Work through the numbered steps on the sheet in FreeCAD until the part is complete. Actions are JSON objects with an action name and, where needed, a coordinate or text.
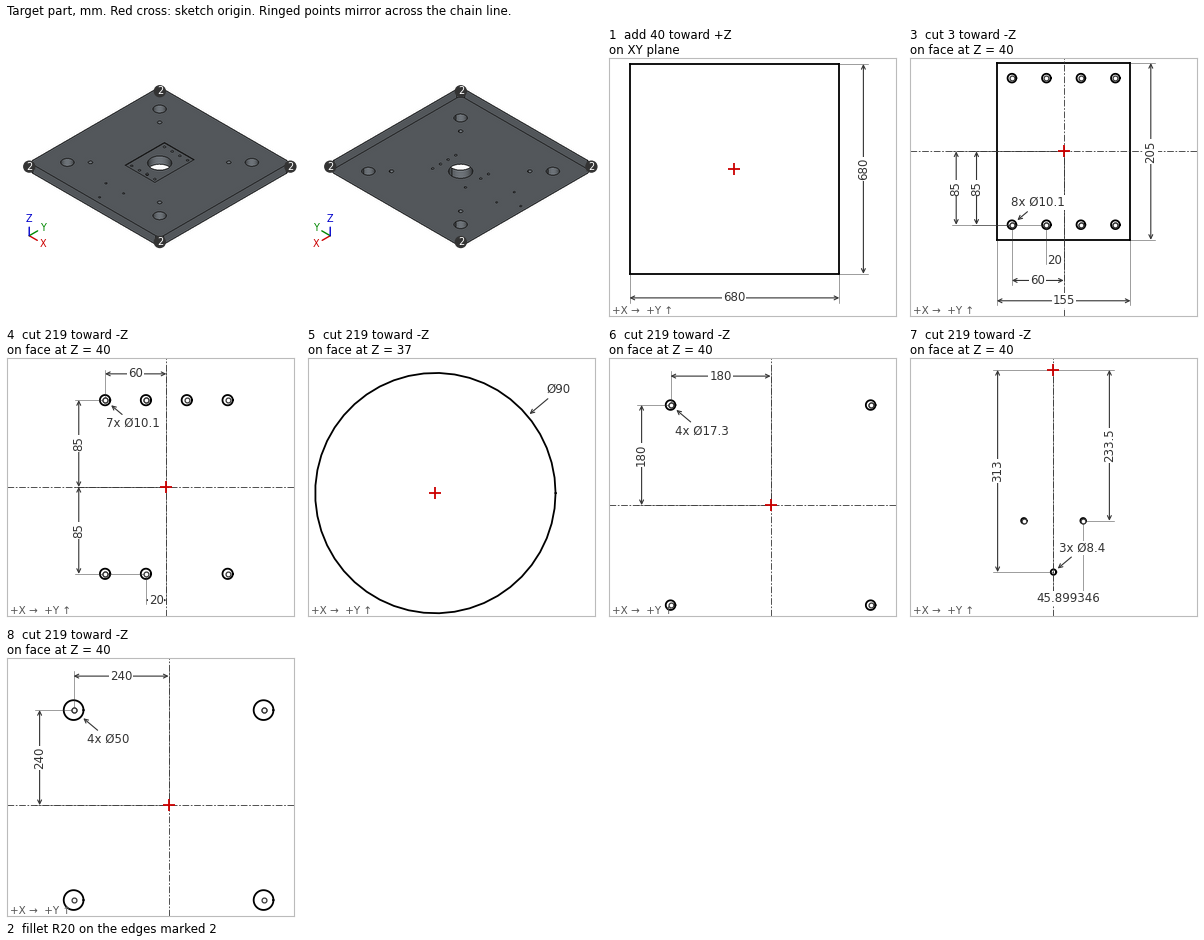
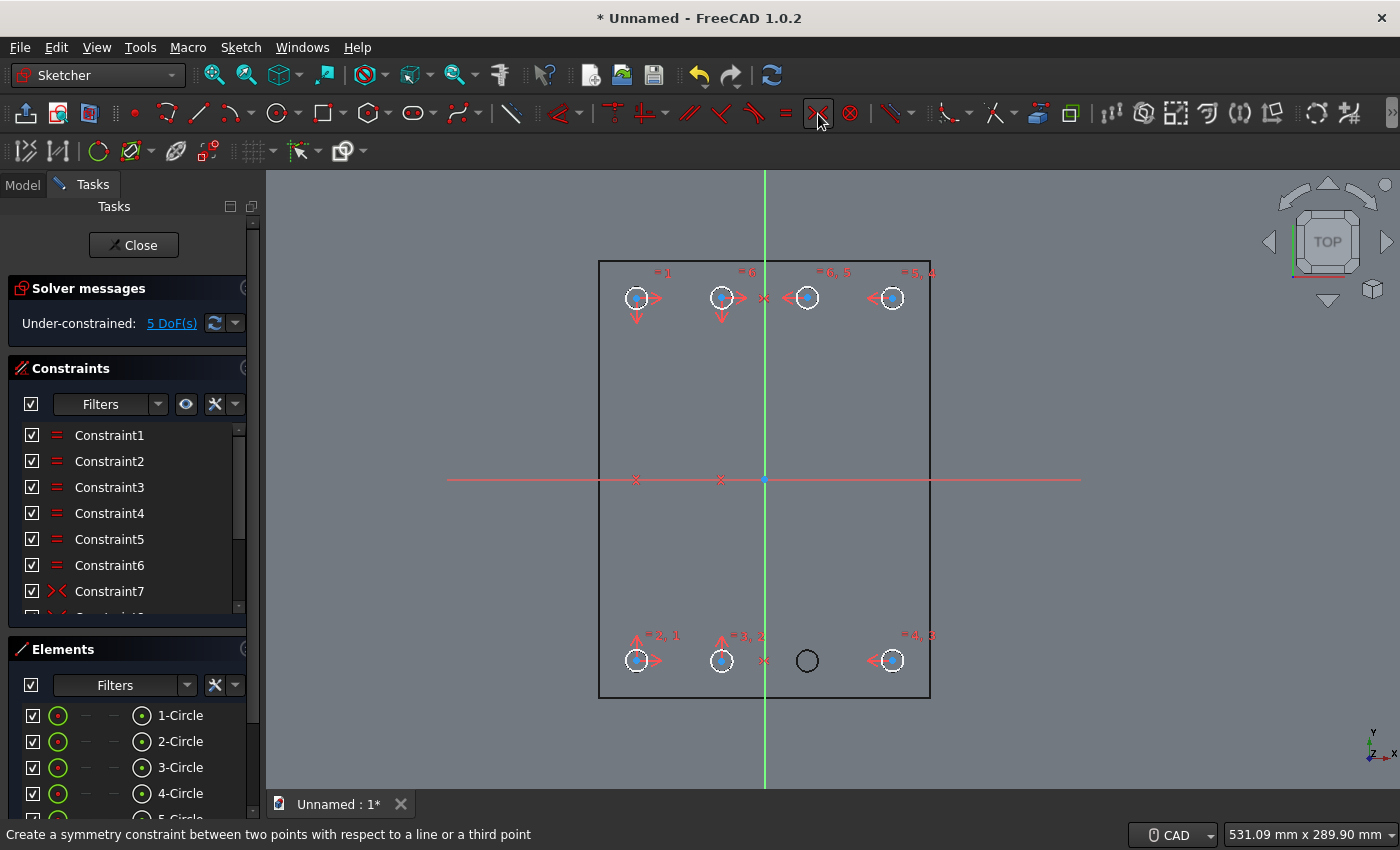
{"action": "left_click", "coordinate": [558, 114]}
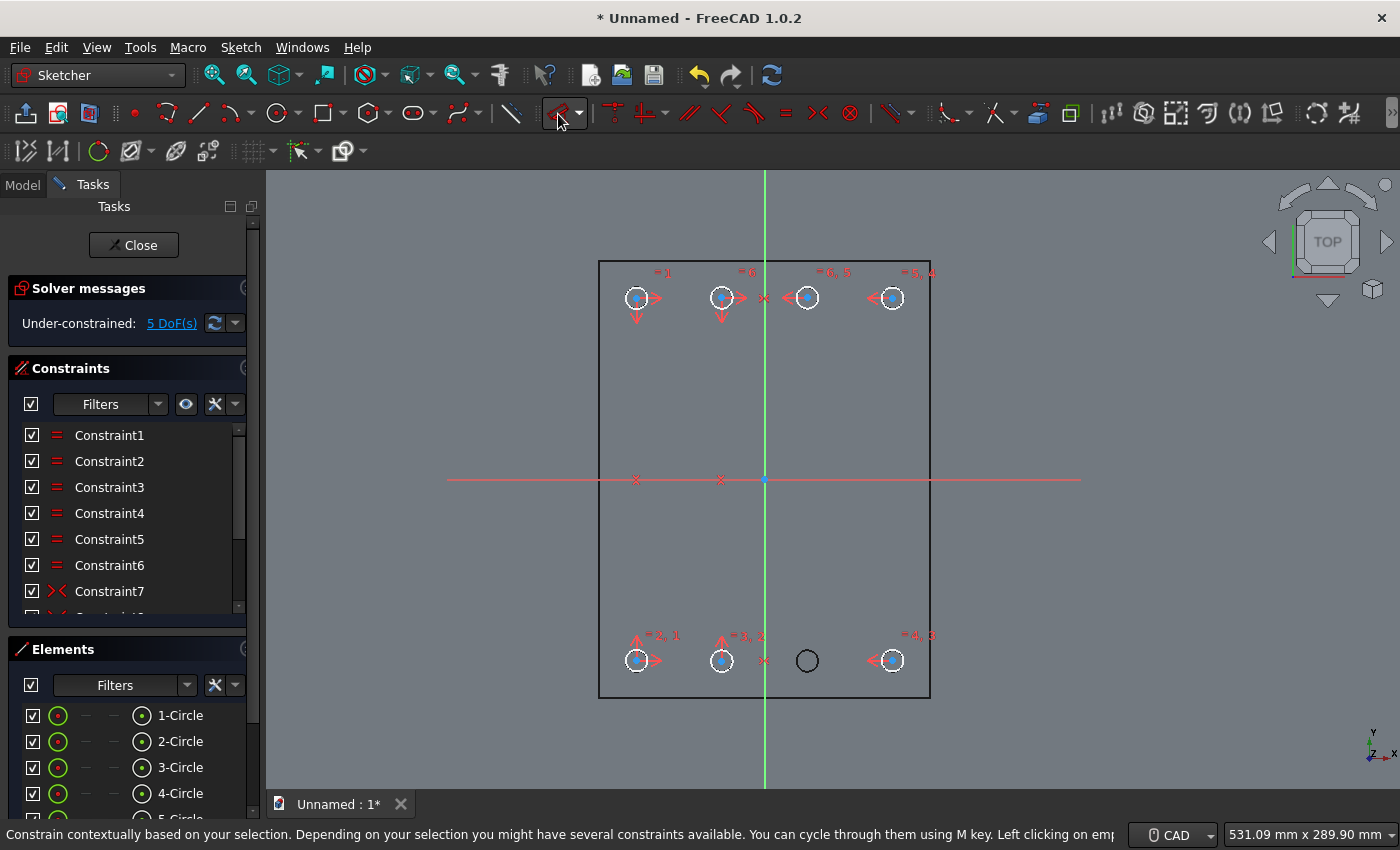
{"action": "scroll", "coordinate": [644, 291], "scroll_direction": "up", "scroll_amount": 4}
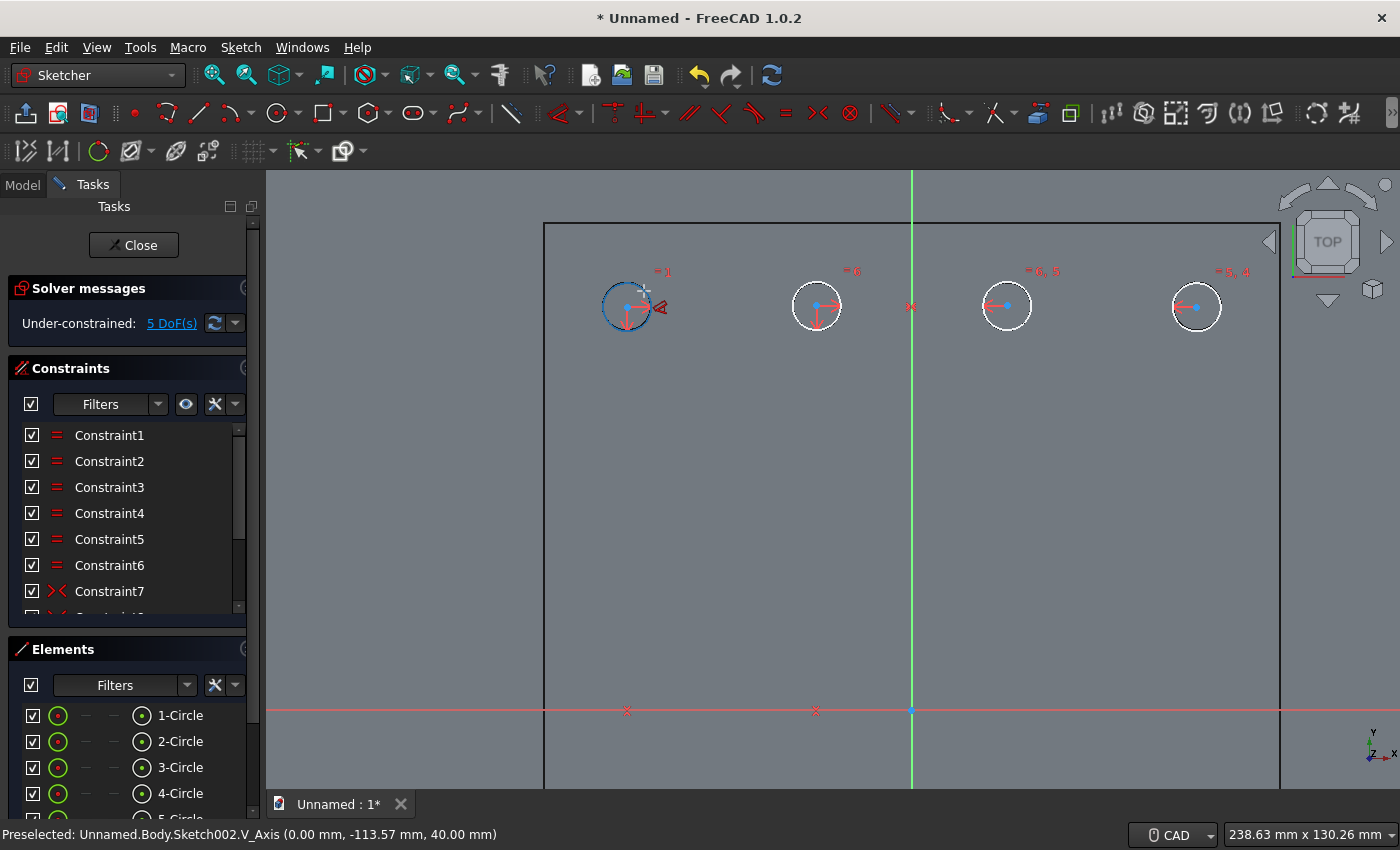
{"action": "left_click", "coordinate": [644, 290]}
{"action": "left_click", "coordinate": [666, 267]}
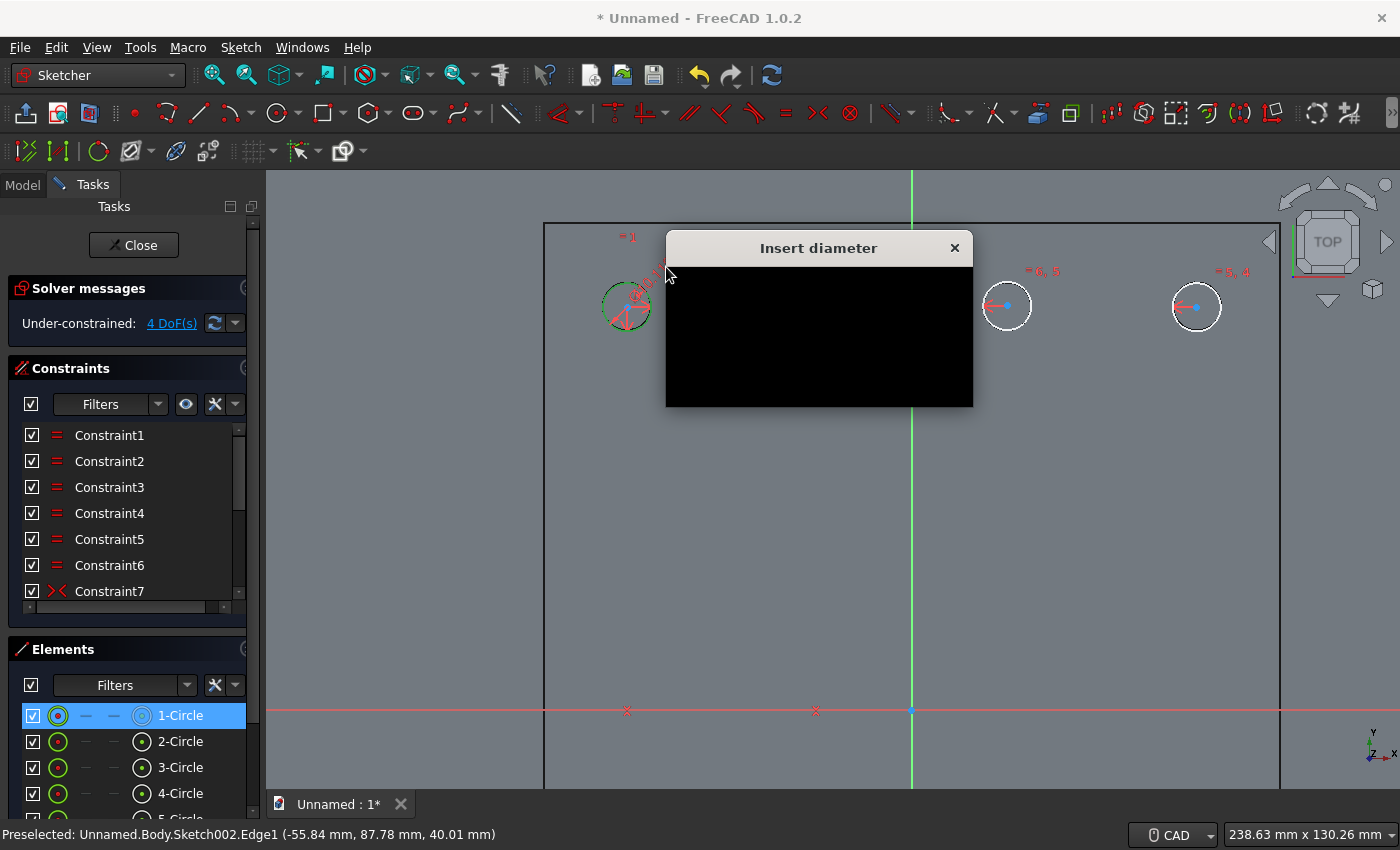
{"action": "type", "text": "10.1"}
{"action": "key", "text": "Return"}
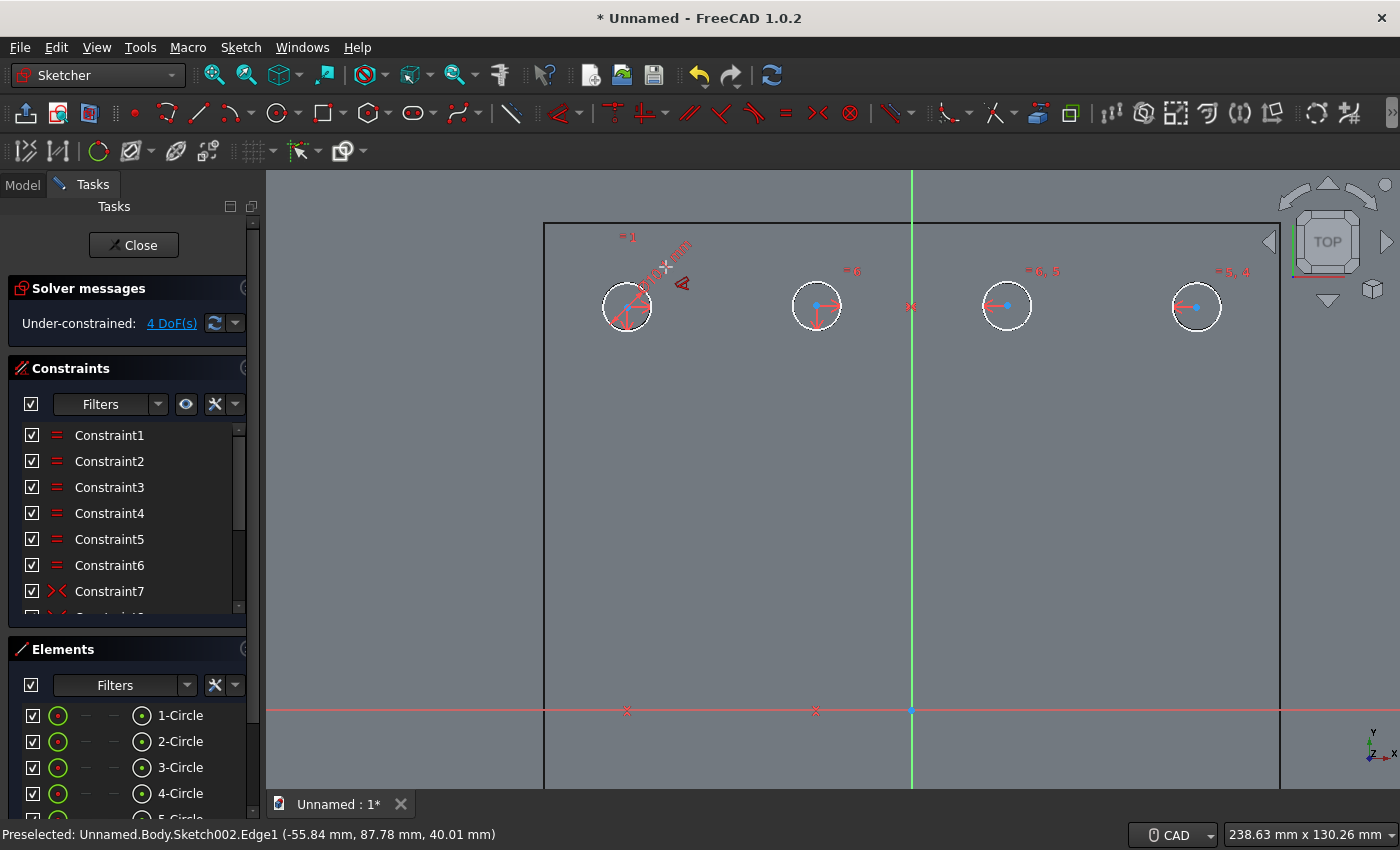
{"action": "left_click", "coordinate": [627, 307]}
{"action": "left_click", "coordinate": [770, 273]}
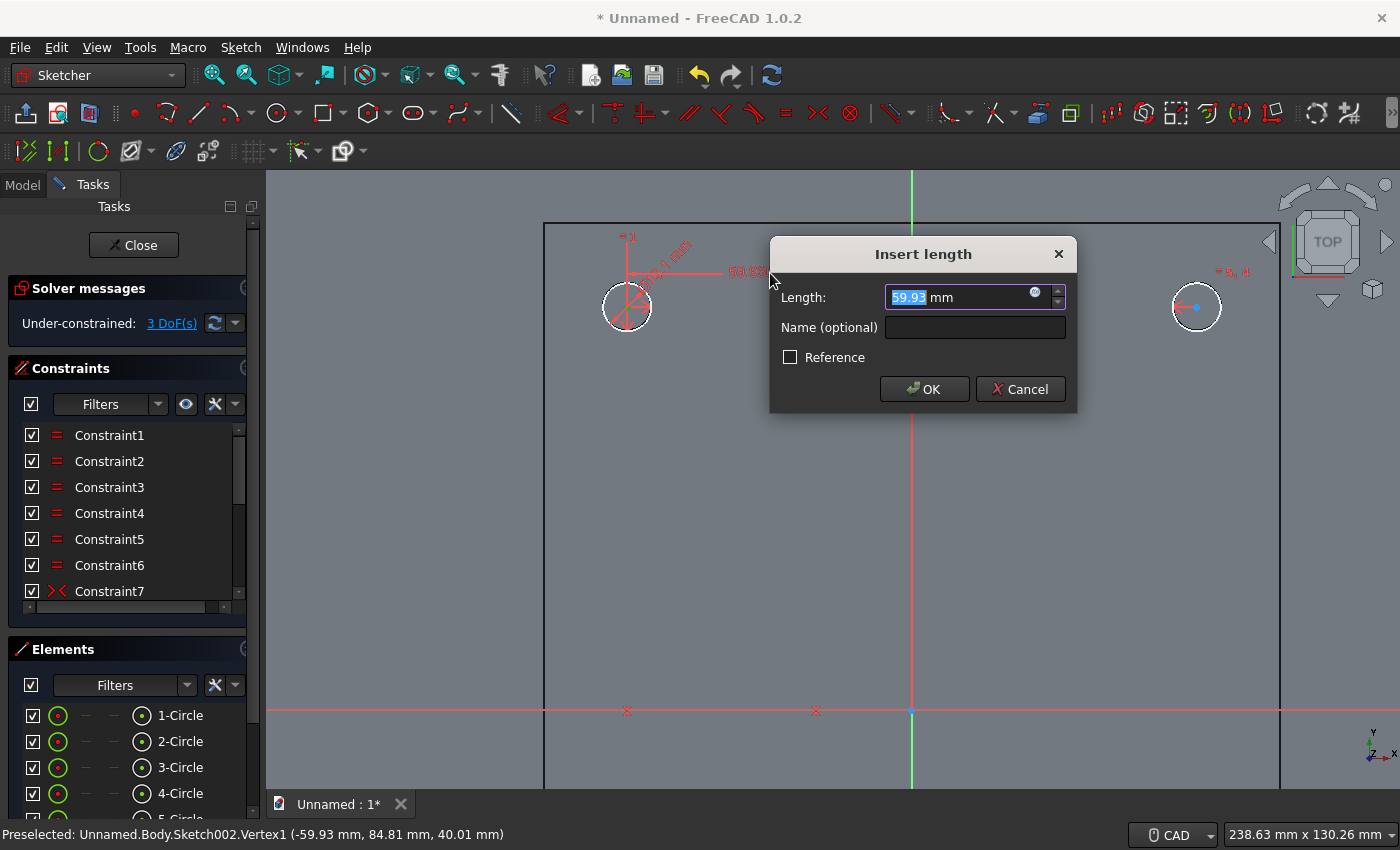
{"action": "type", "text": "60"}
{"action": "key", "text": "Return"}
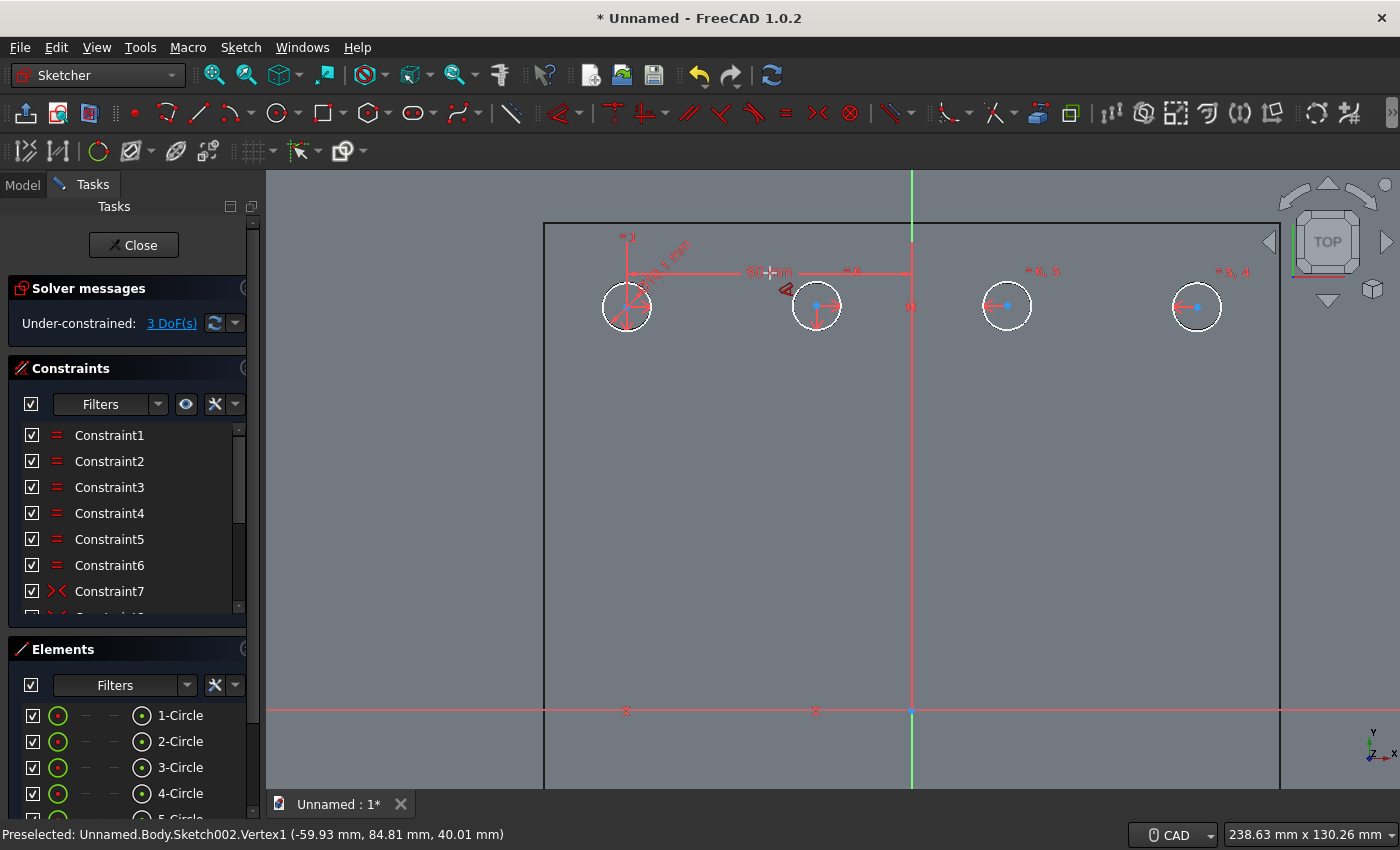
{"action": "left_click", "coordinate": [627, 307]}
{"action": "left_click", "coordinate": [593, 509]}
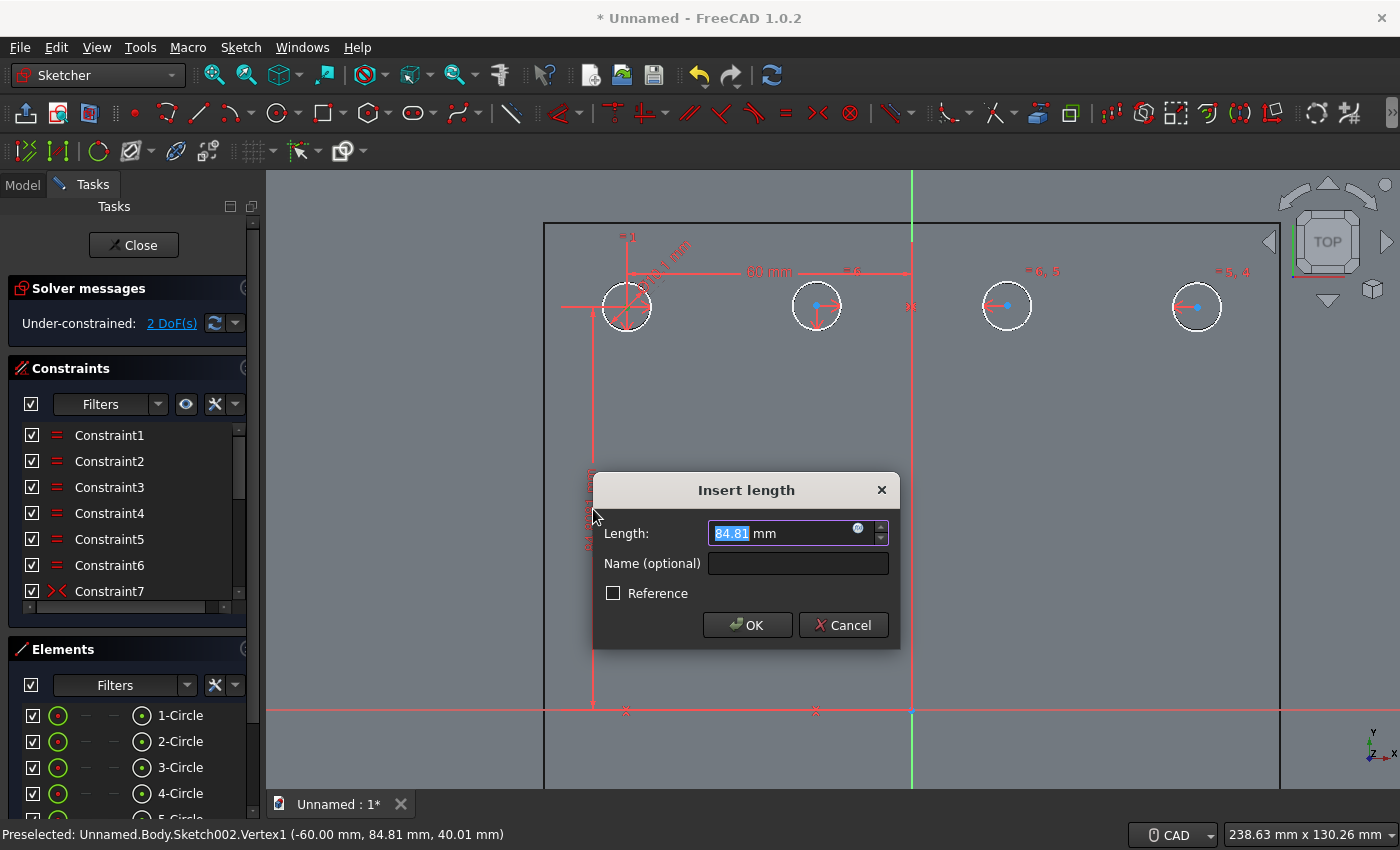
{"action": "type", "text": "85"}
{"action": "key", "text": "Return"}